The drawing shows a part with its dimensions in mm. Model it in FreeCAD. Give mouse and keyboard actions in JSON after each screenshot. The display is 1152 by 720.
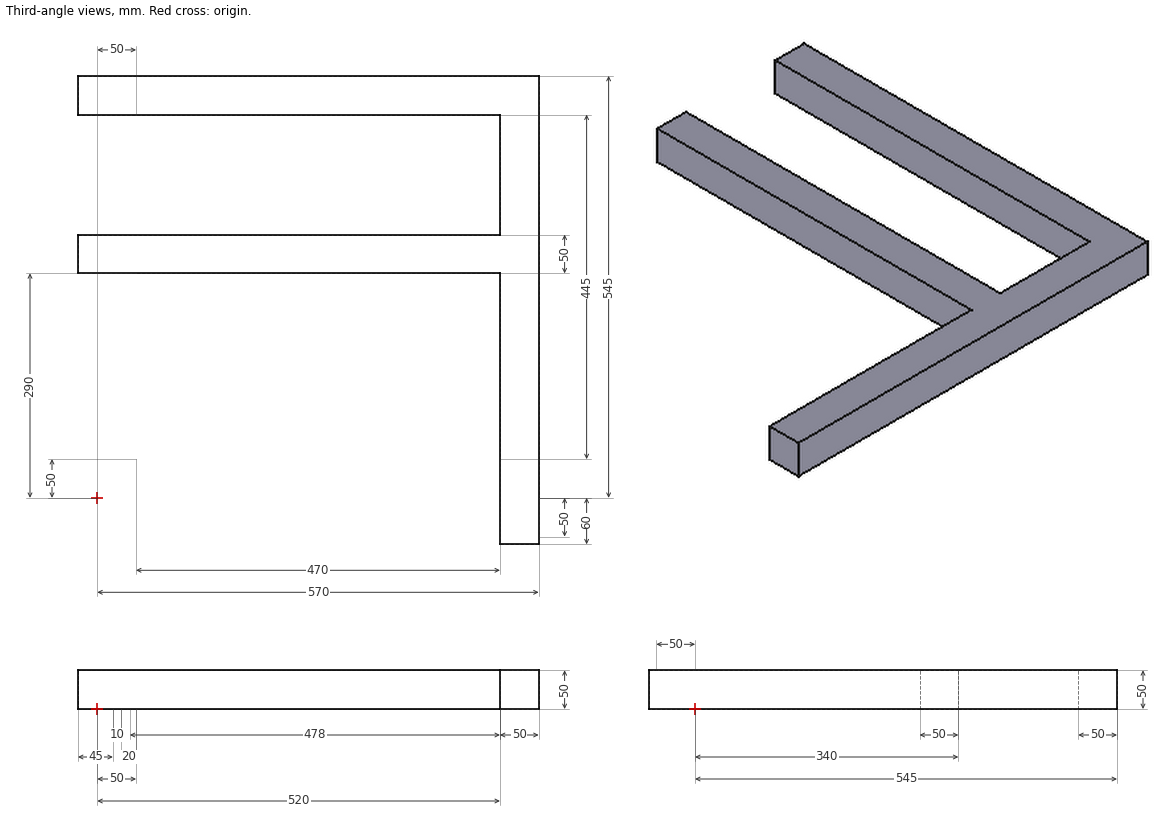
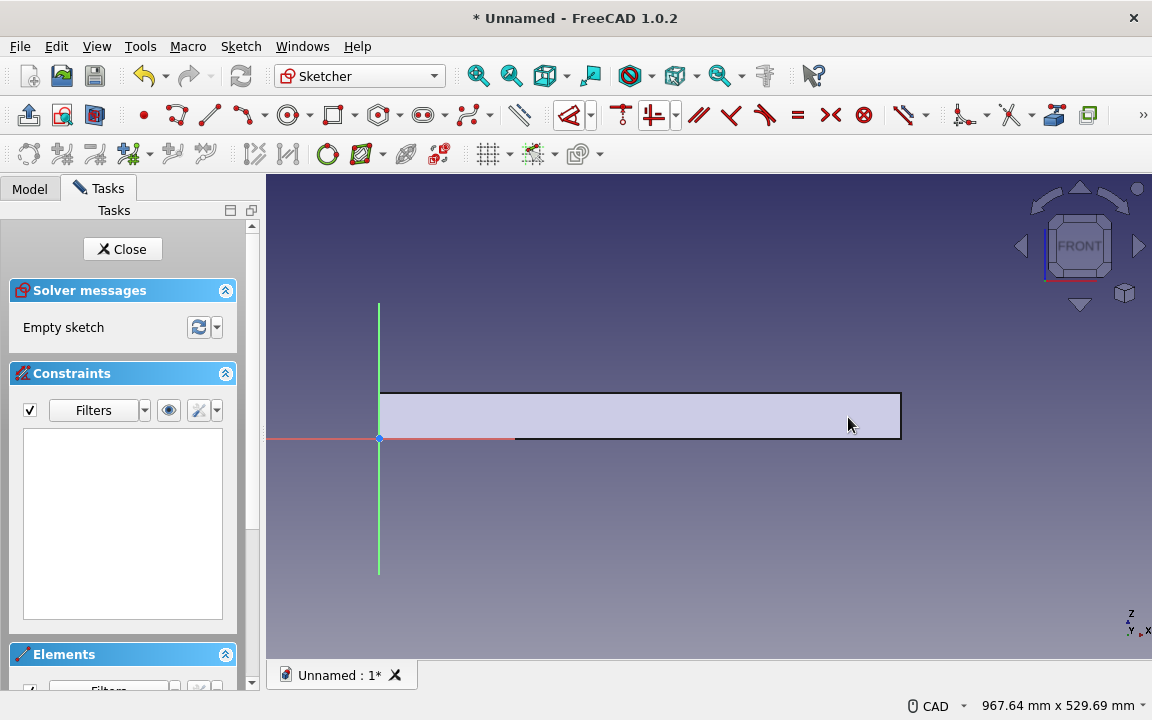
{"action": "key", "text": "g r"}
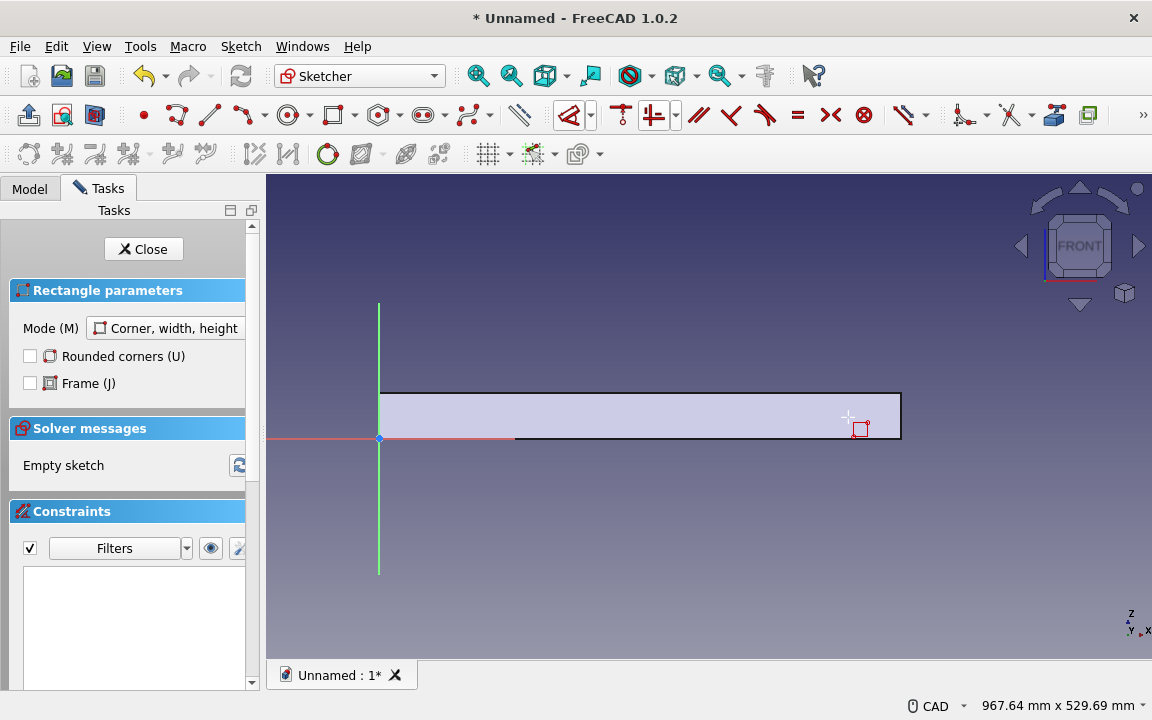
{"action": "left_click", "coordinate": [379, 439]}
{"action": "mouse_move", "coordinate": [425, 393]}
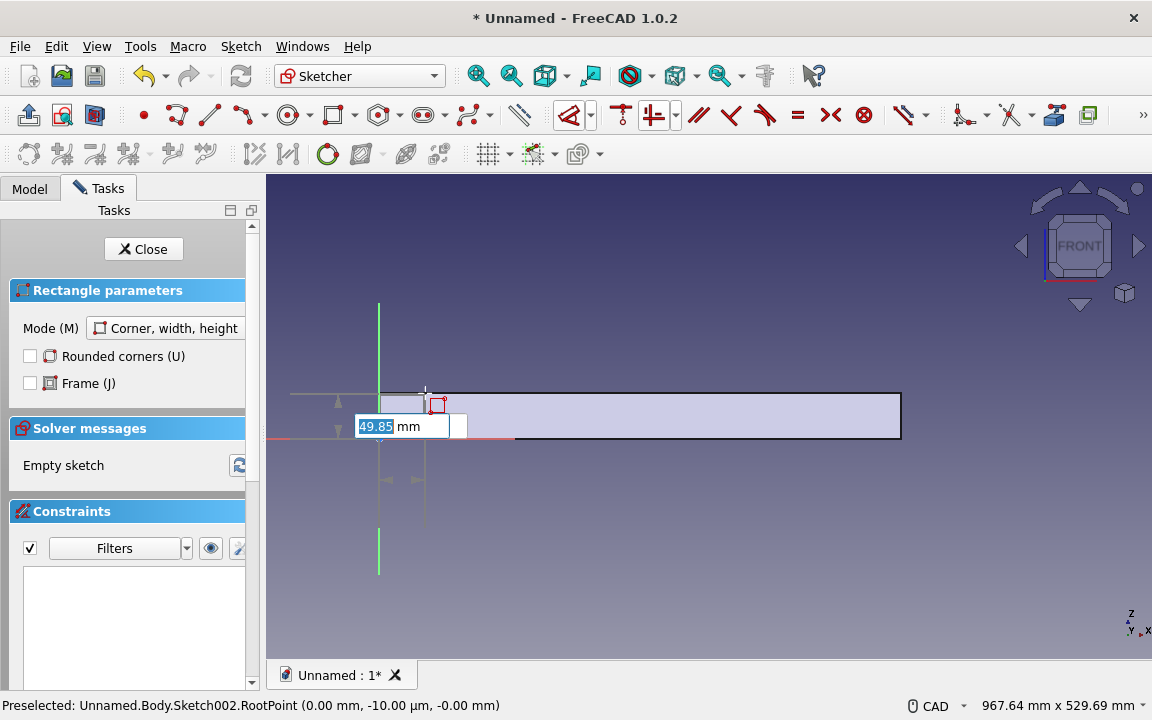
{"action": "type", "text": "50"}
{"action": "key", "text": "Tab"}
{"action": "type", "text": "50"}
{"action": "key", "text": "Return"}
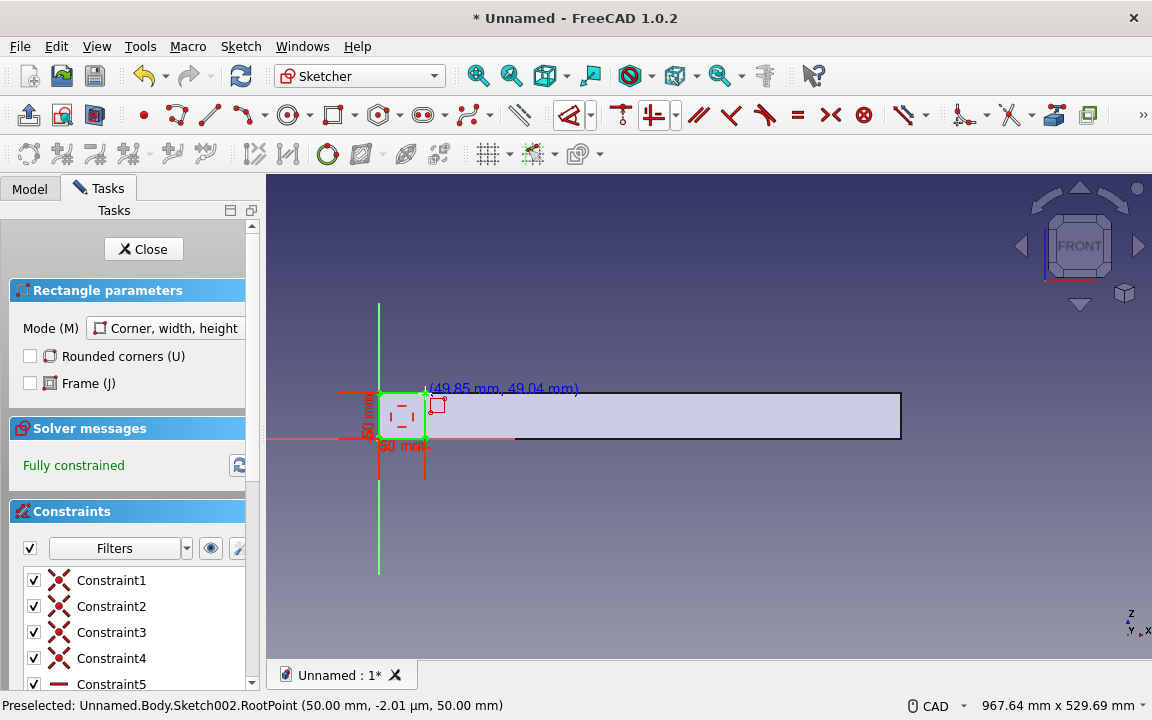
{"action": "left_click", "coordinate": [855, 393]}
{"action": "left_click", "coordinate": [901, 439]}
{"action": "key", "text": "Escape"}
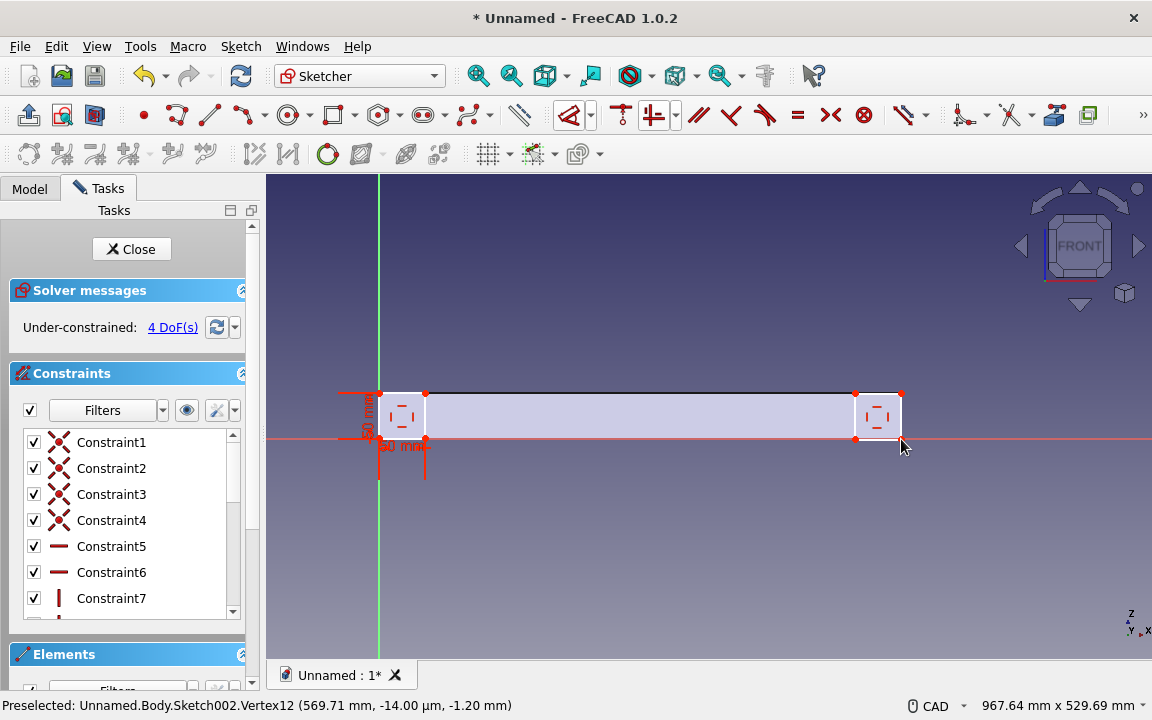
{"action": "left_click", "coordinate": [855, 440]}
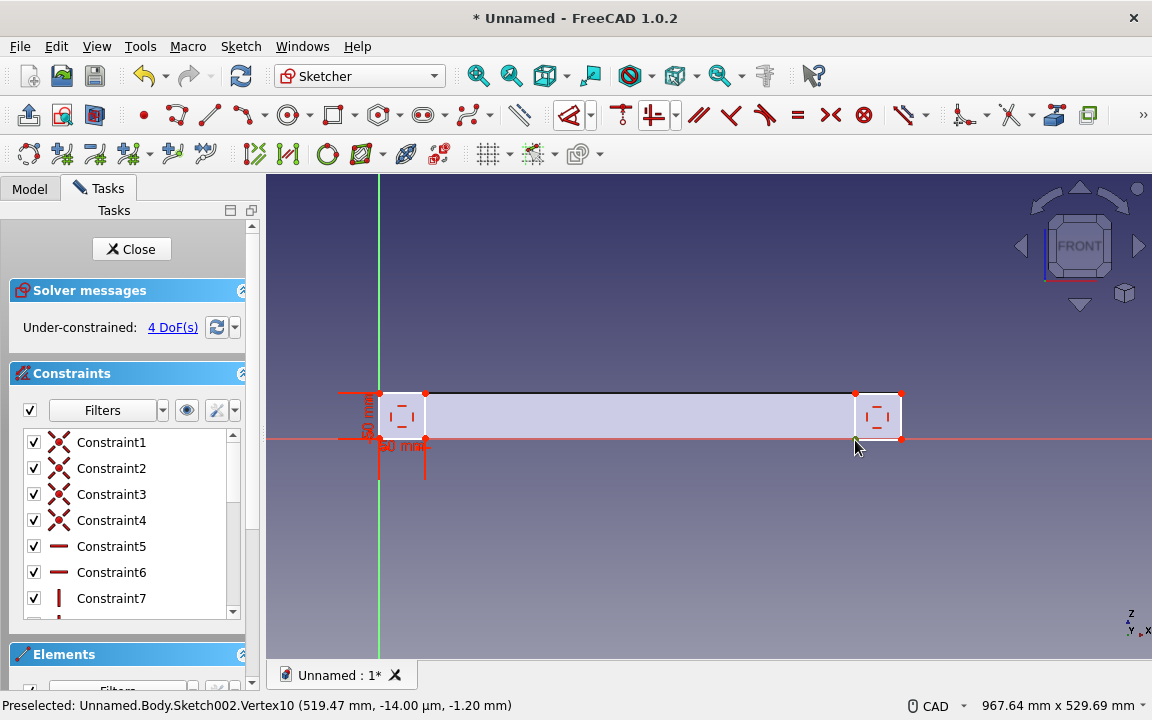
{"action": "left_click", "coordinate": [344, 439]}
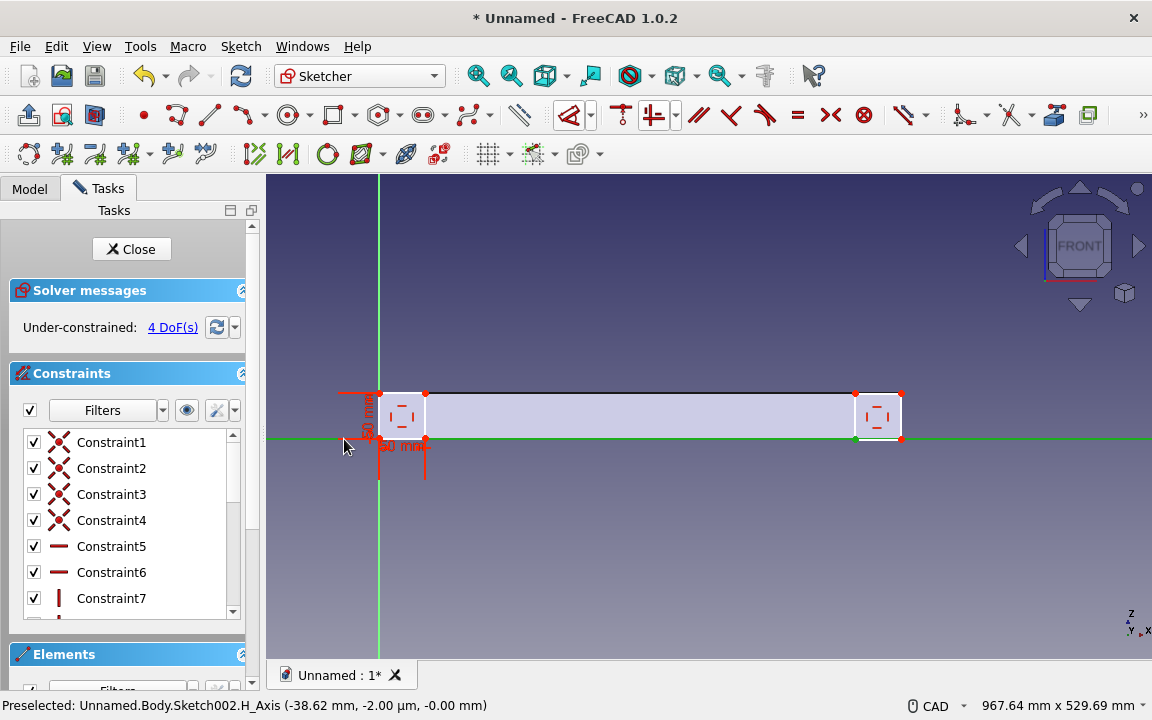
{"action": "key", "text": "c"}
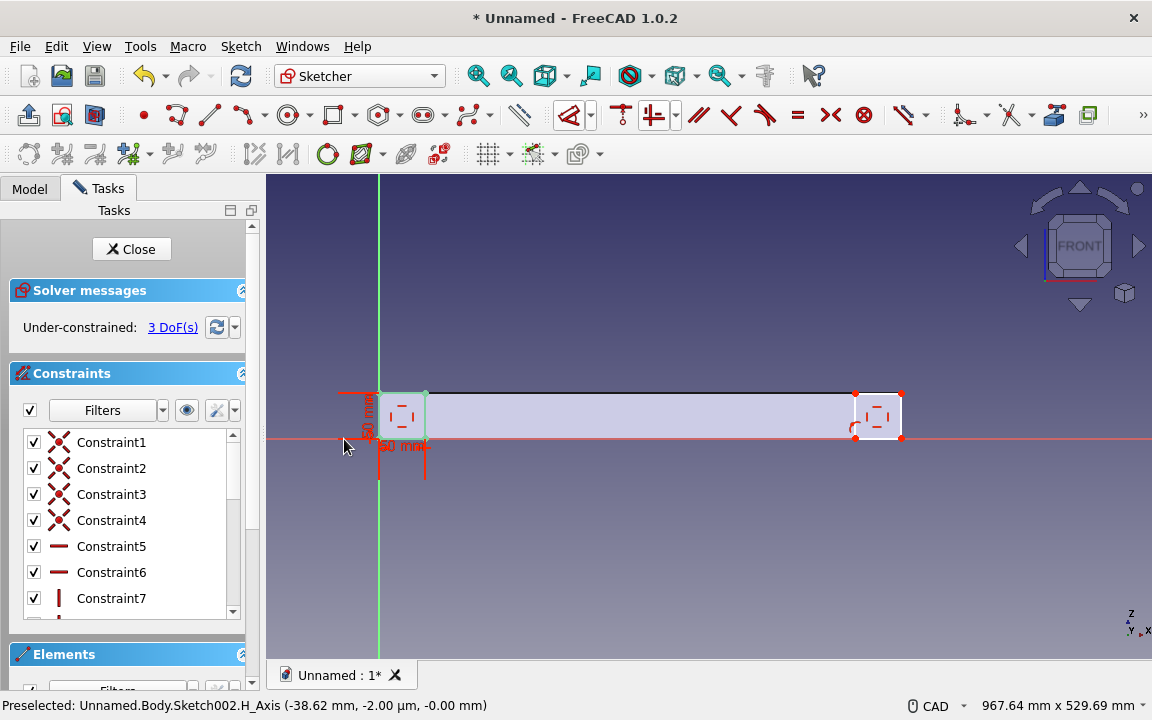
{"action": "left_click", "coordinate": [855, 407]}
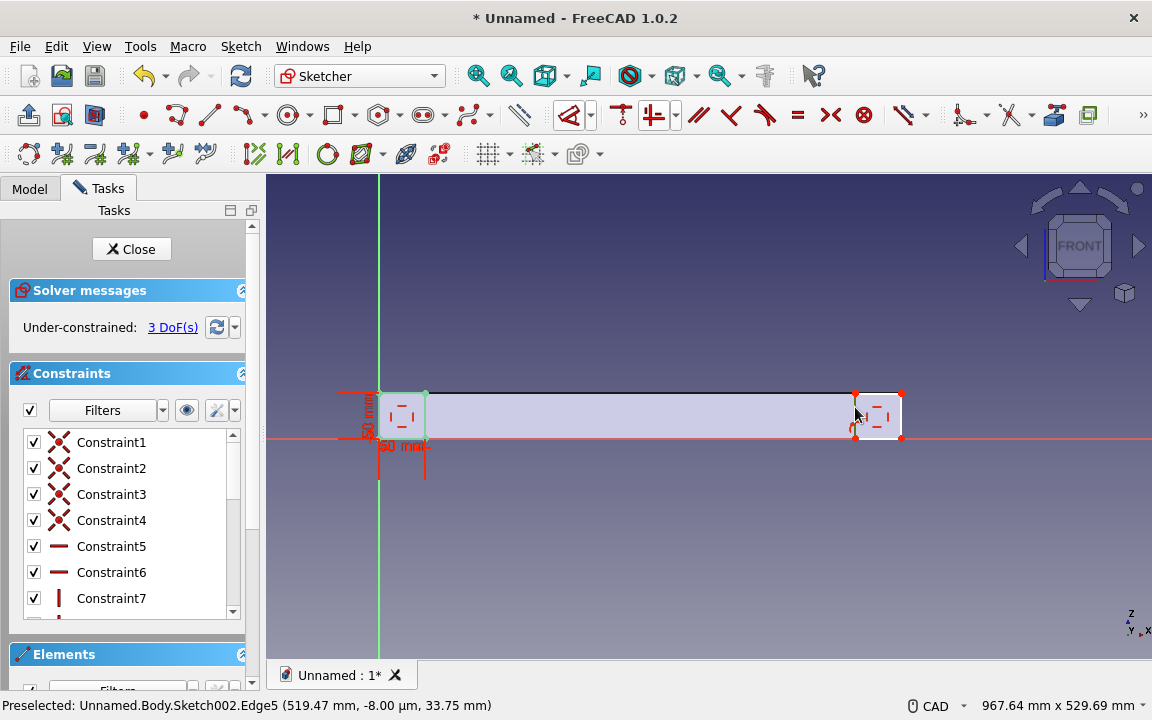
{"action": "key", "text": "i"}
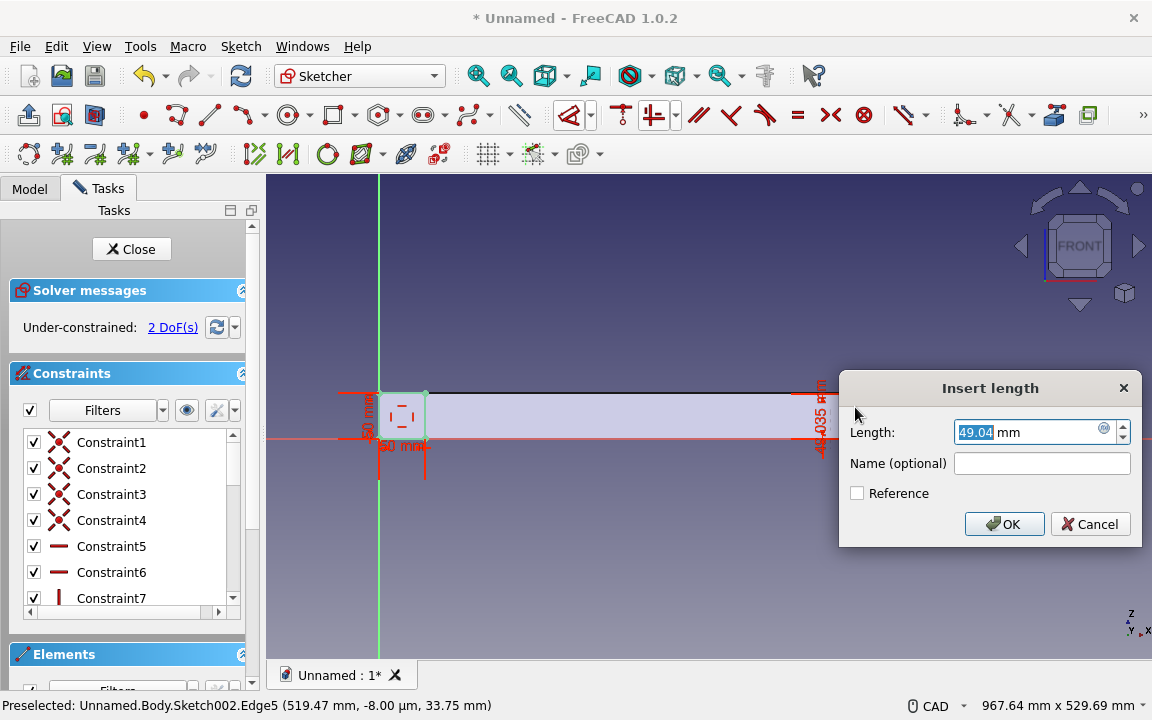
{"action": "type", "text": "50"}
{"action": "key", "text": "Return"}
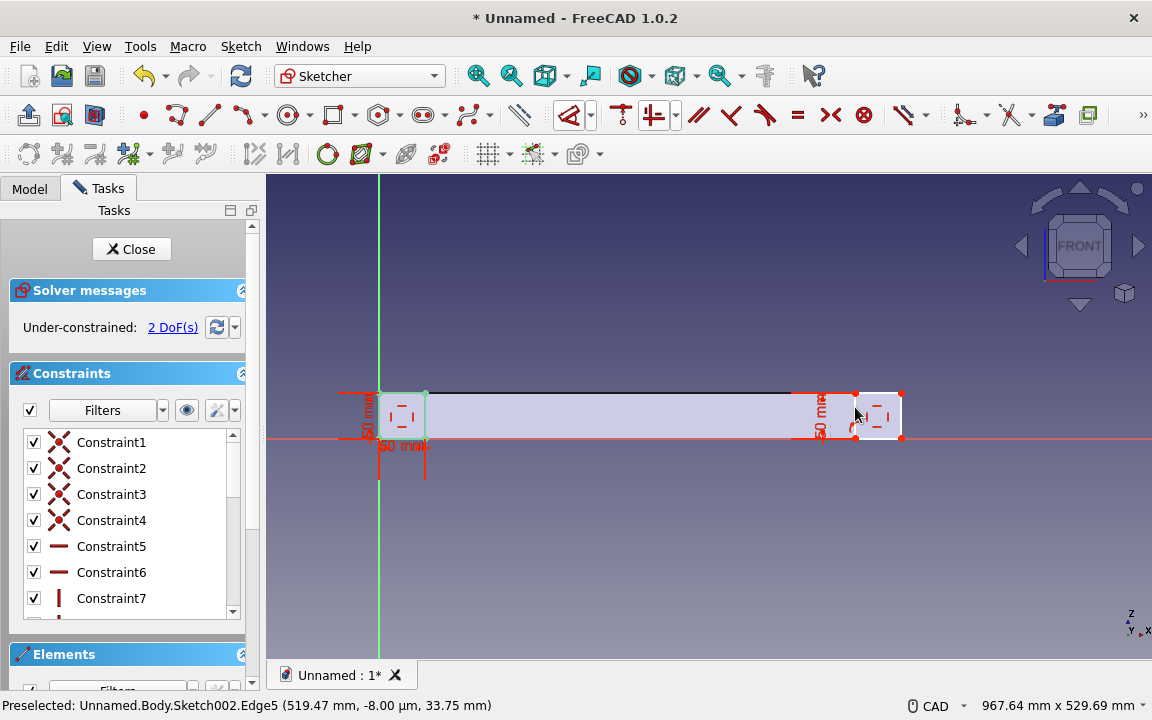
{"action": "left_click", "coordinate": [869, 439]}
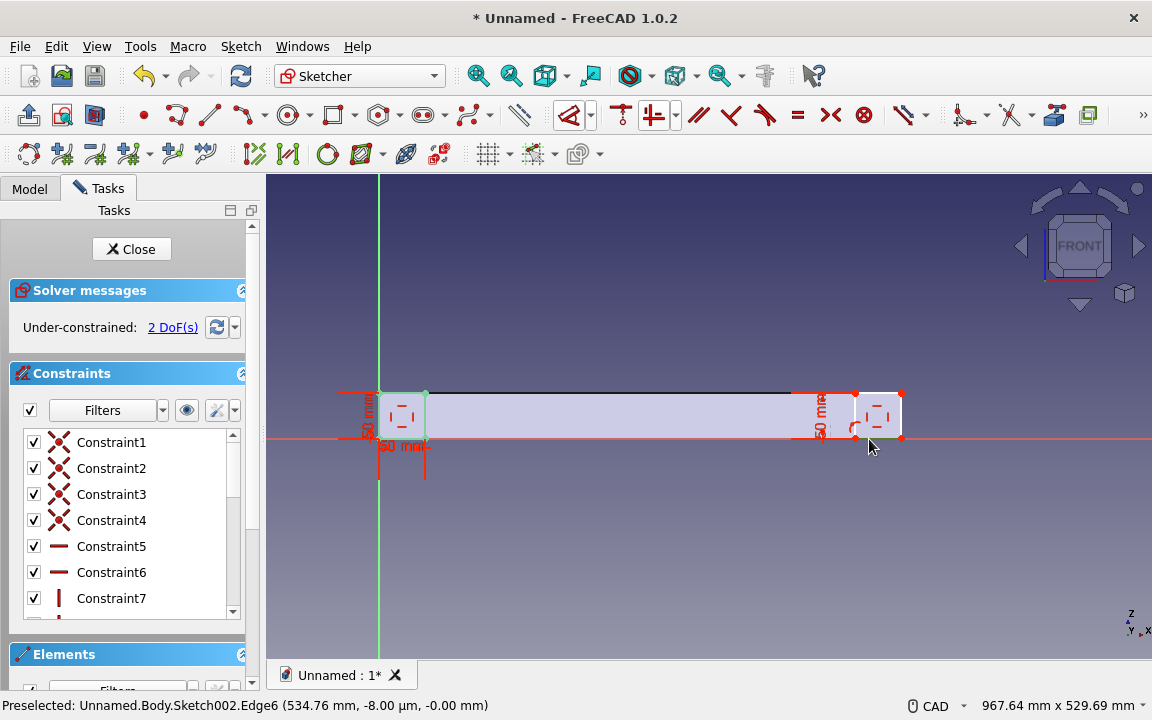
{"action": "key", "text": "l"}